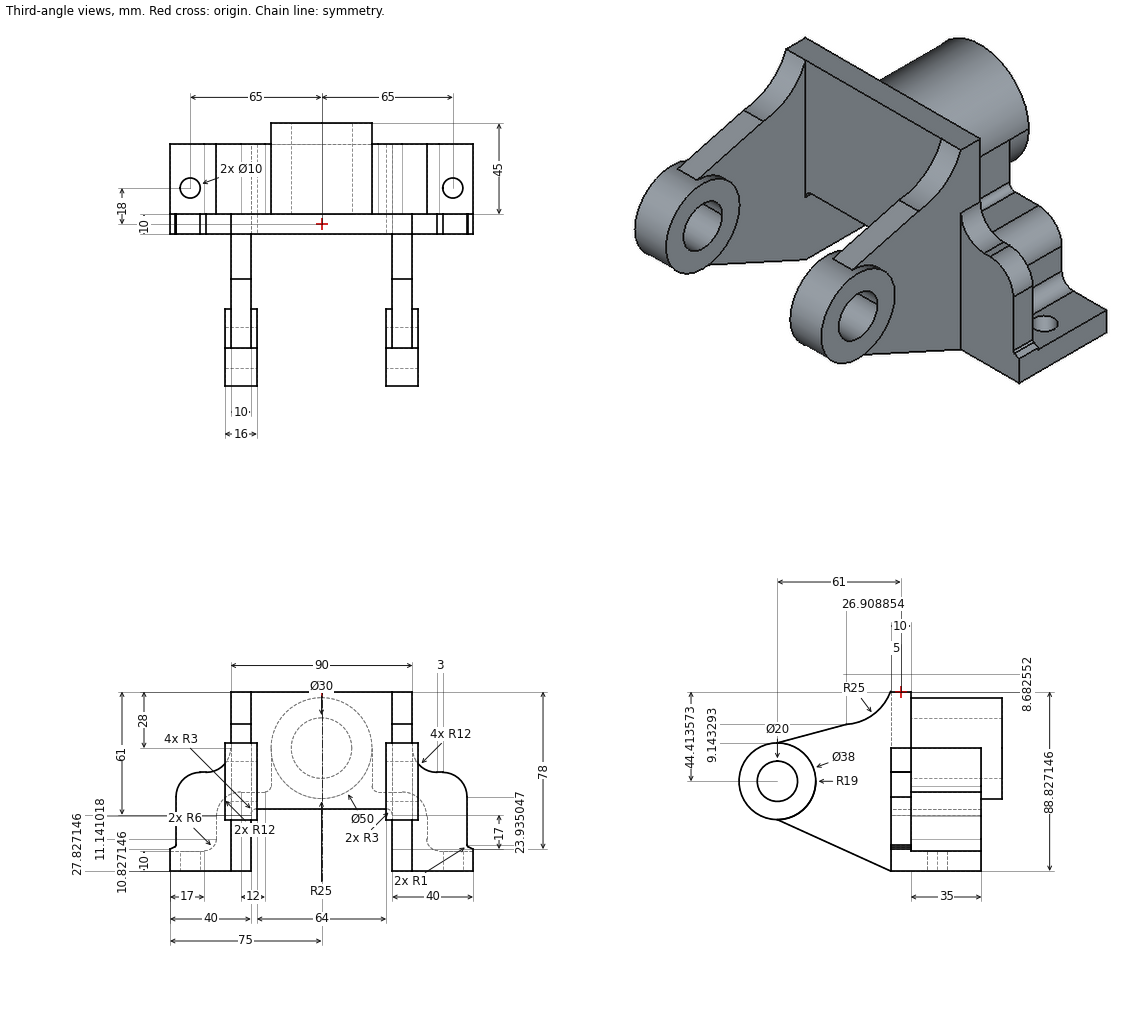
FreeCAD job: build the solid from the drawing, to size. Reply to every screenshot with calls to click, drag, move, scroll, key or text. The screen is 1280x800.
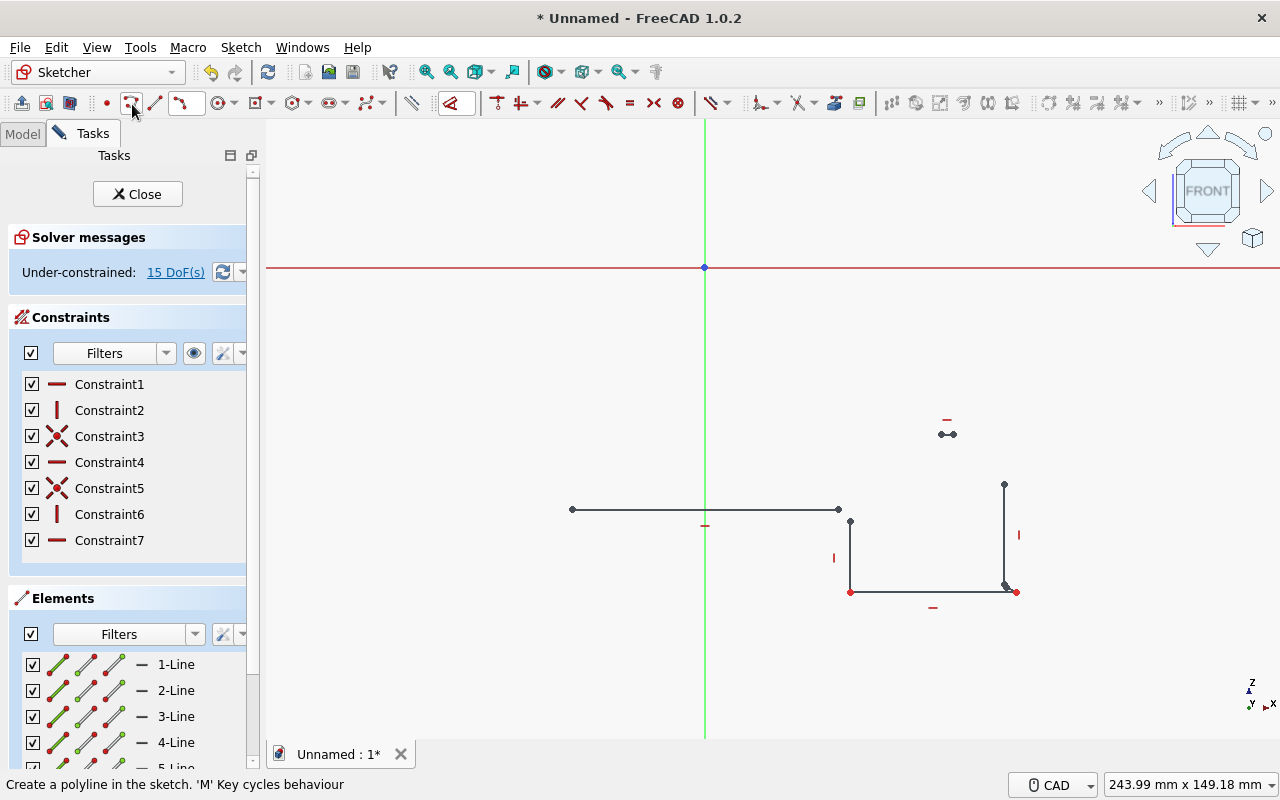
click(559, 521)
click(559, 592)
click(393, 592)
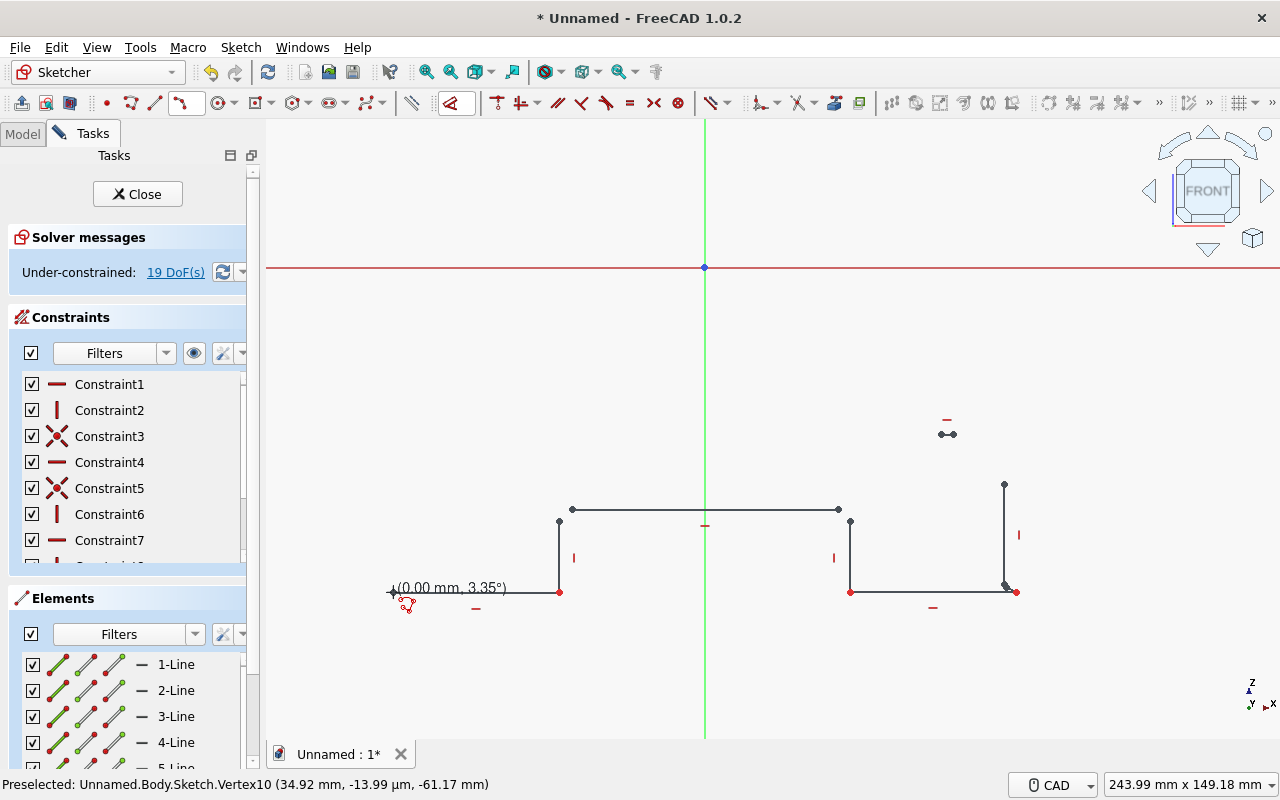
scroll(403, 587, up, 6)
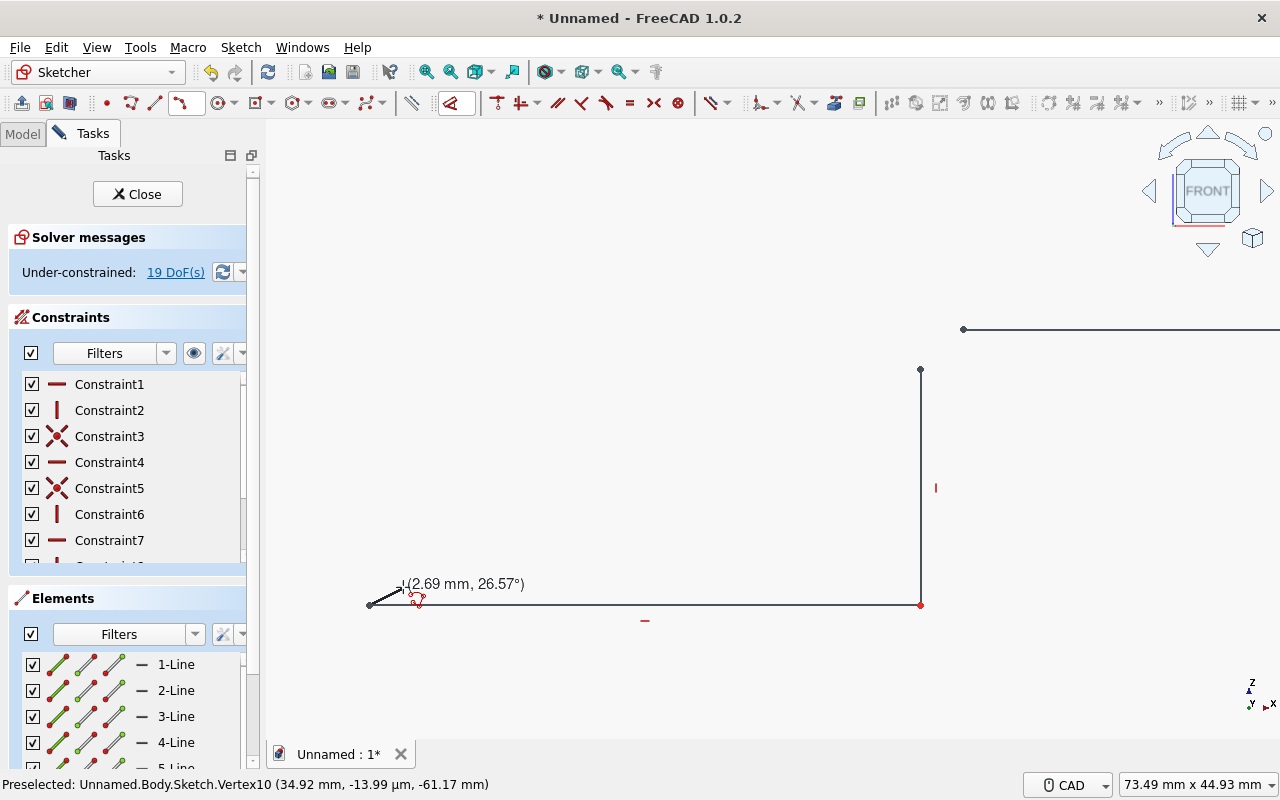
click(404, 586)
right_click(404, 586)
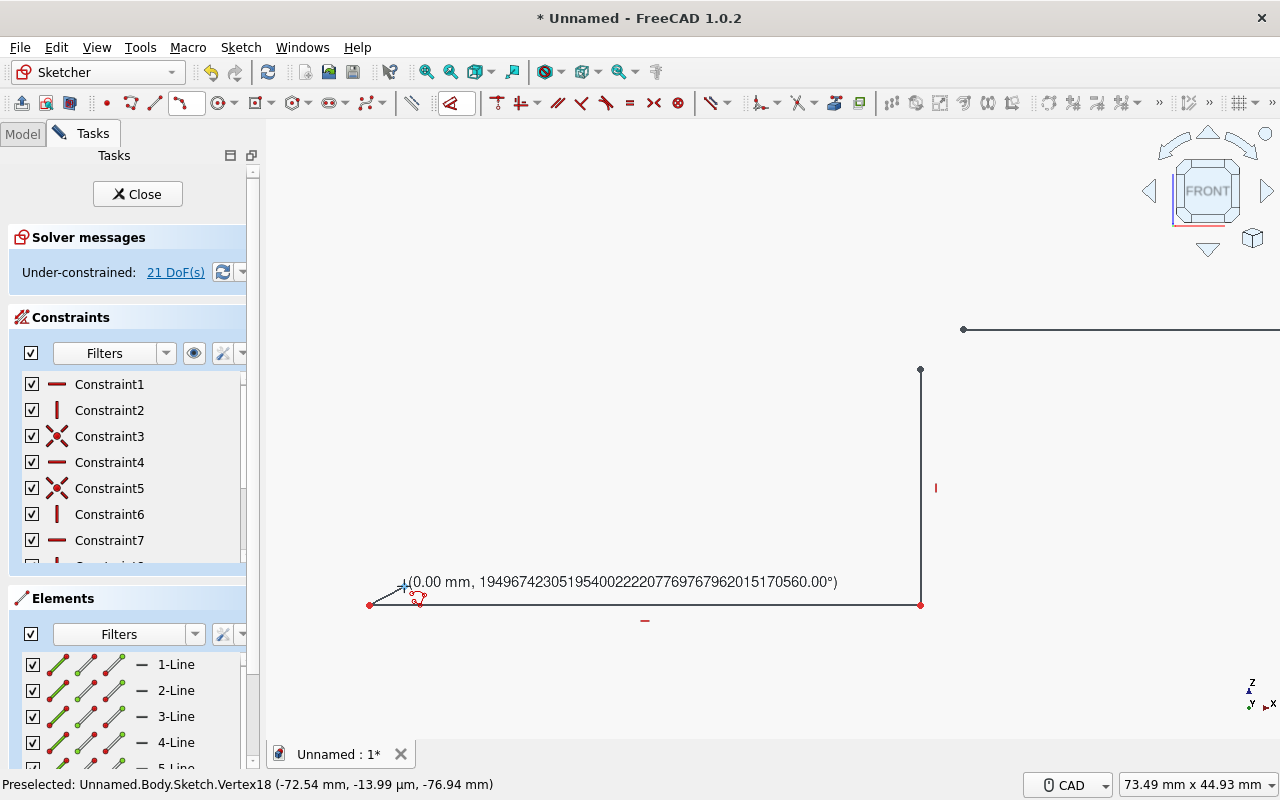
key(g)
key(l)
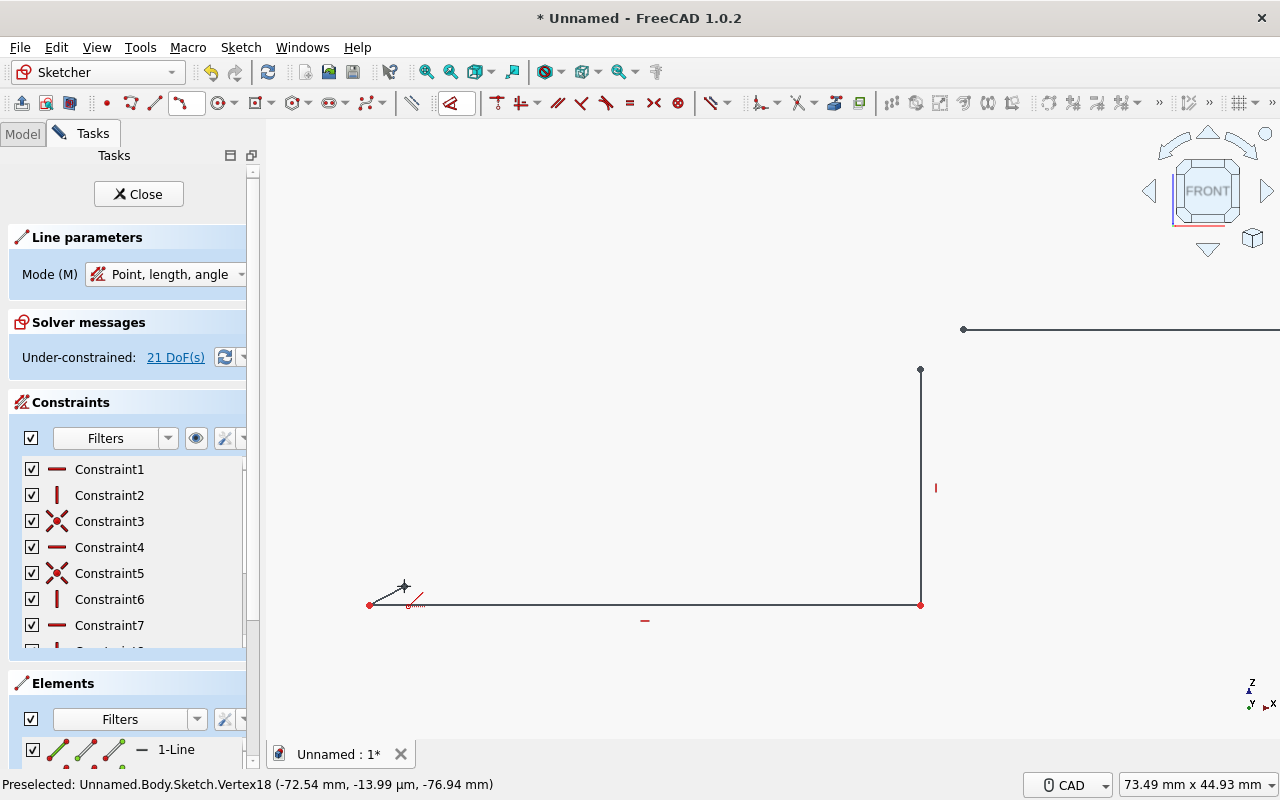
click(411, 573)
click(411, 243)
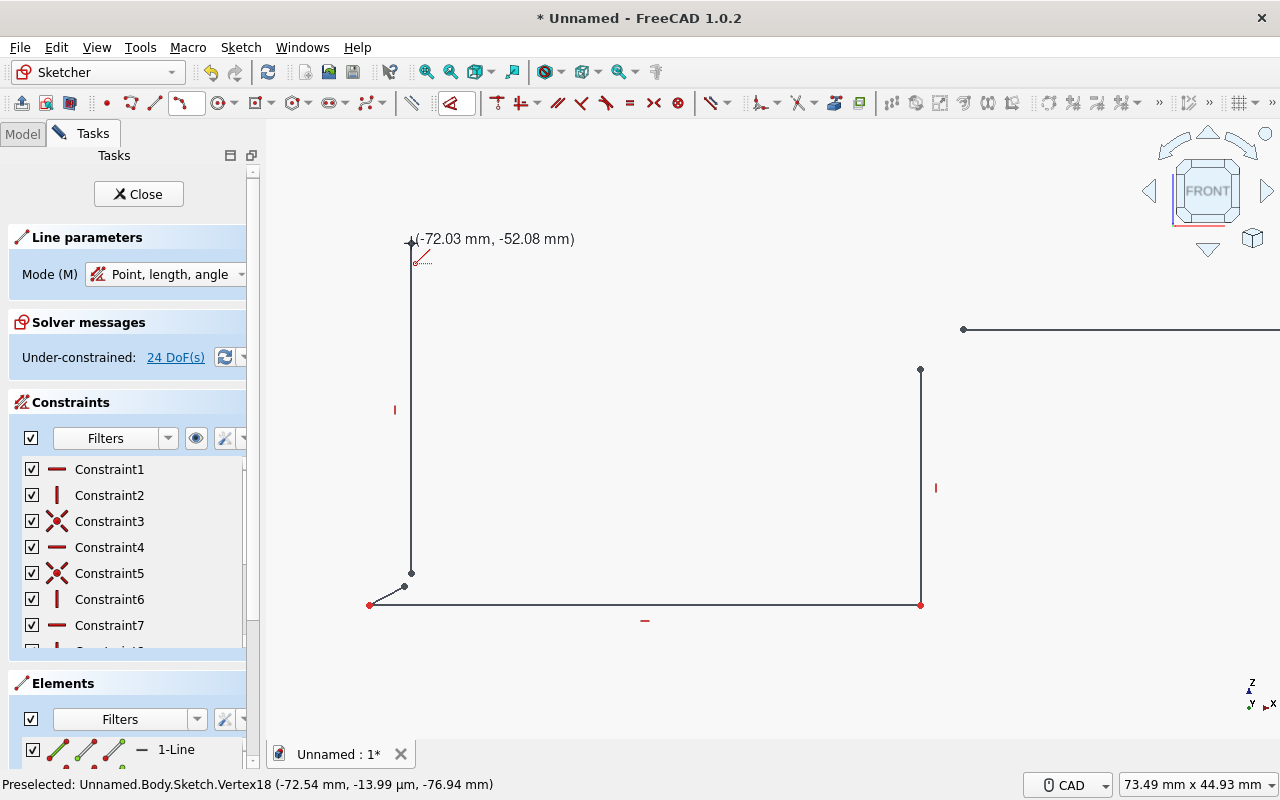
scroll(403, 587, down, 6)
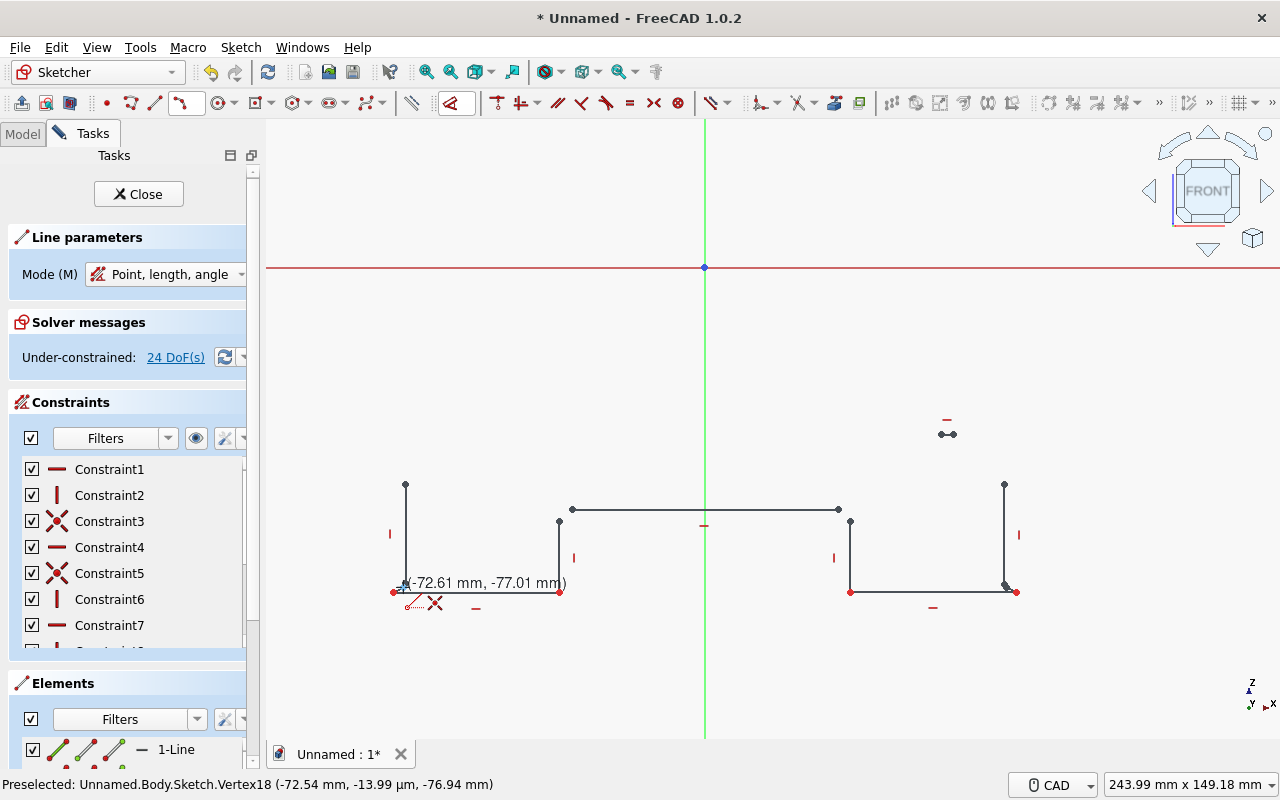
click(455, 434)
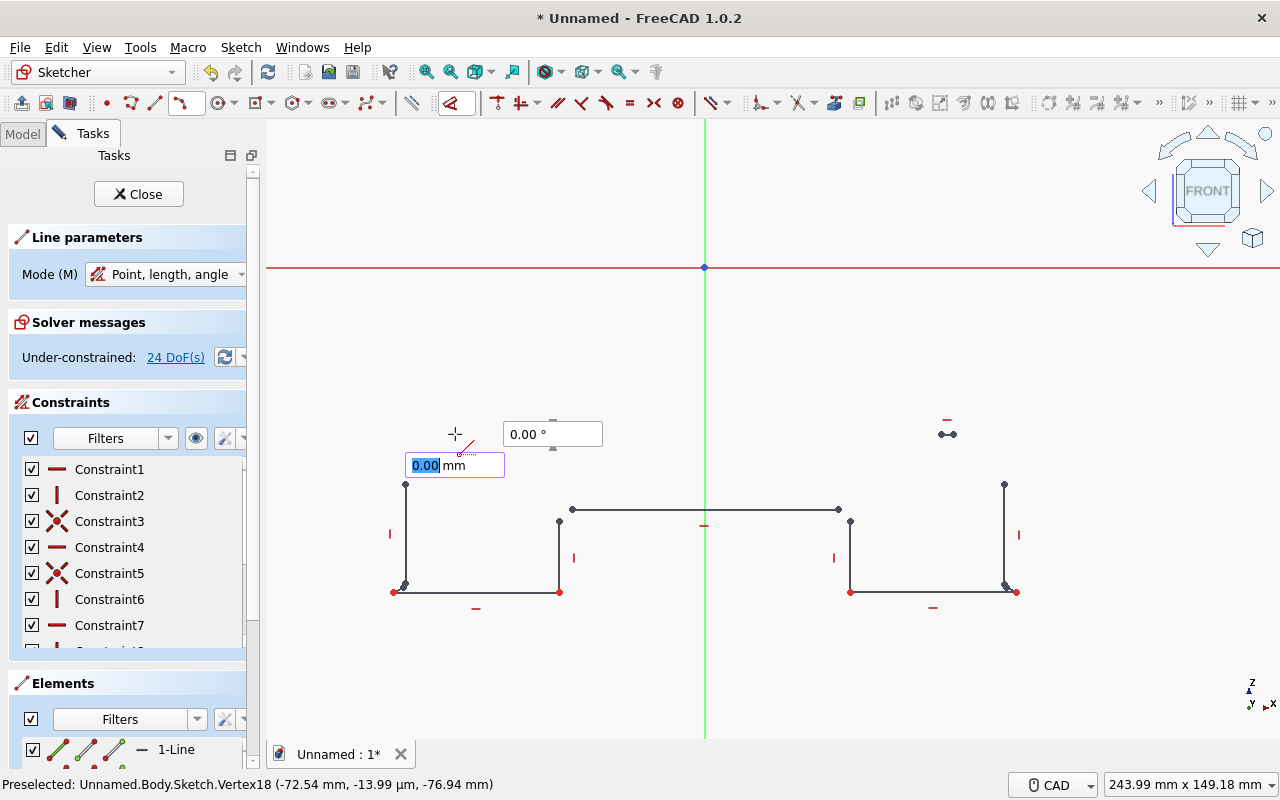
scroll(468, 434, up, 2)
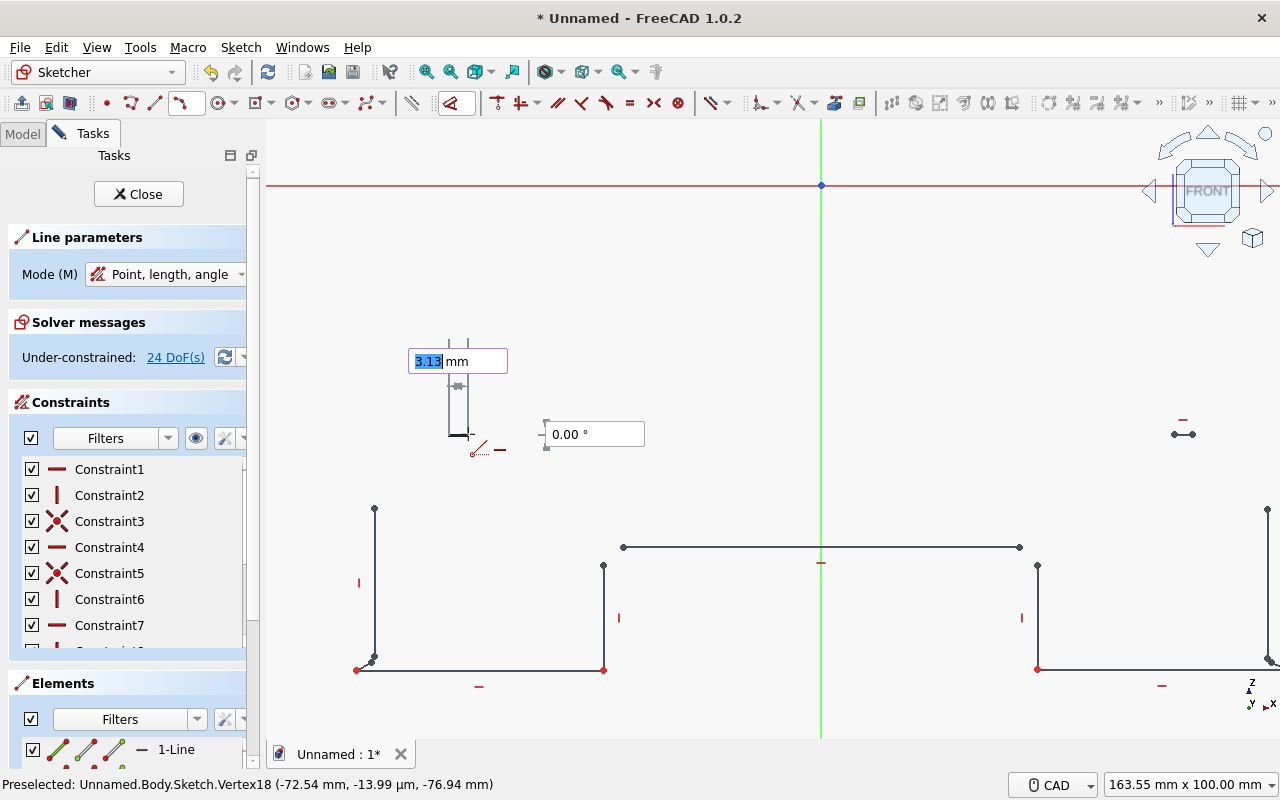
click(468, 434)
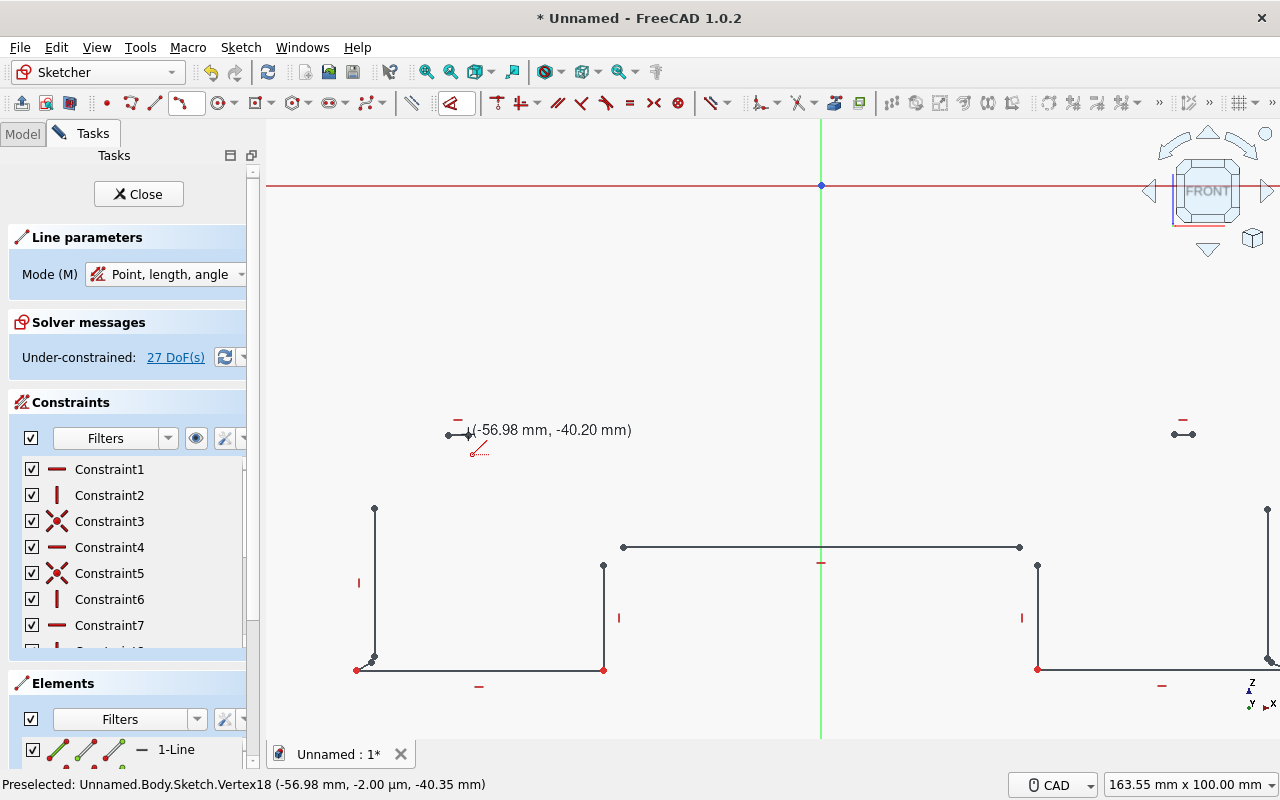
key(g)
key(m)